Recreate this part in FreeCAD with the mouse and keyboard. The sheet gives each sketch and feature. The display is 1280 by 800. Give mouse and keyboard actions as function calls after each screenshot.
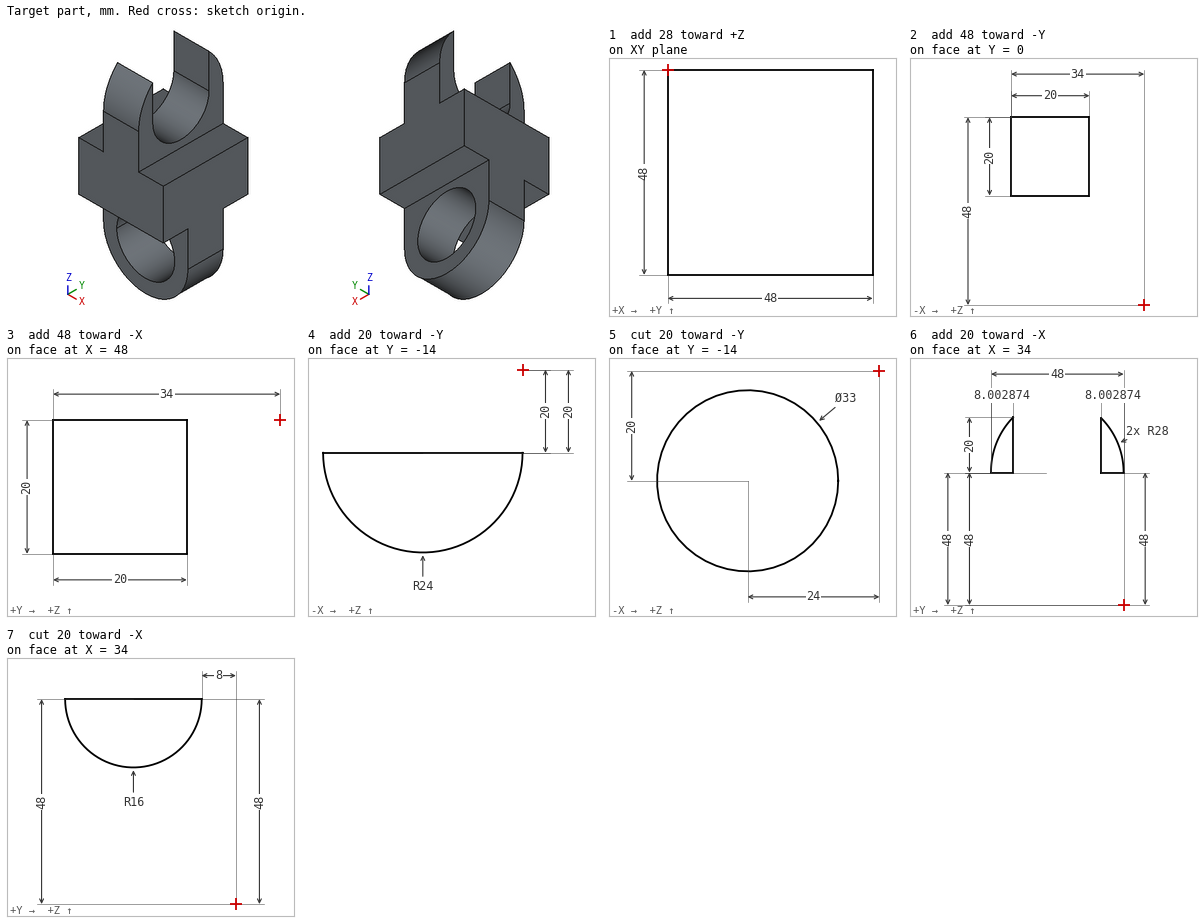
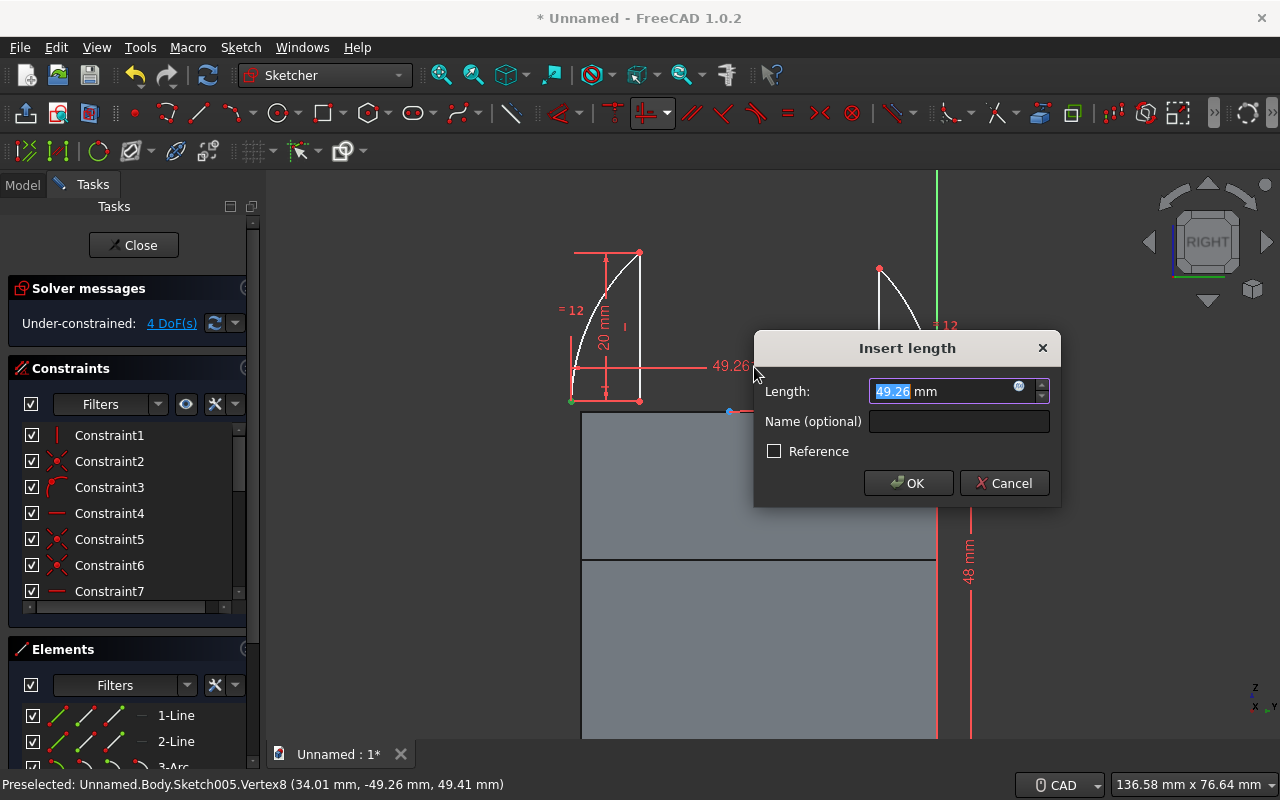
text(48)
key(Return)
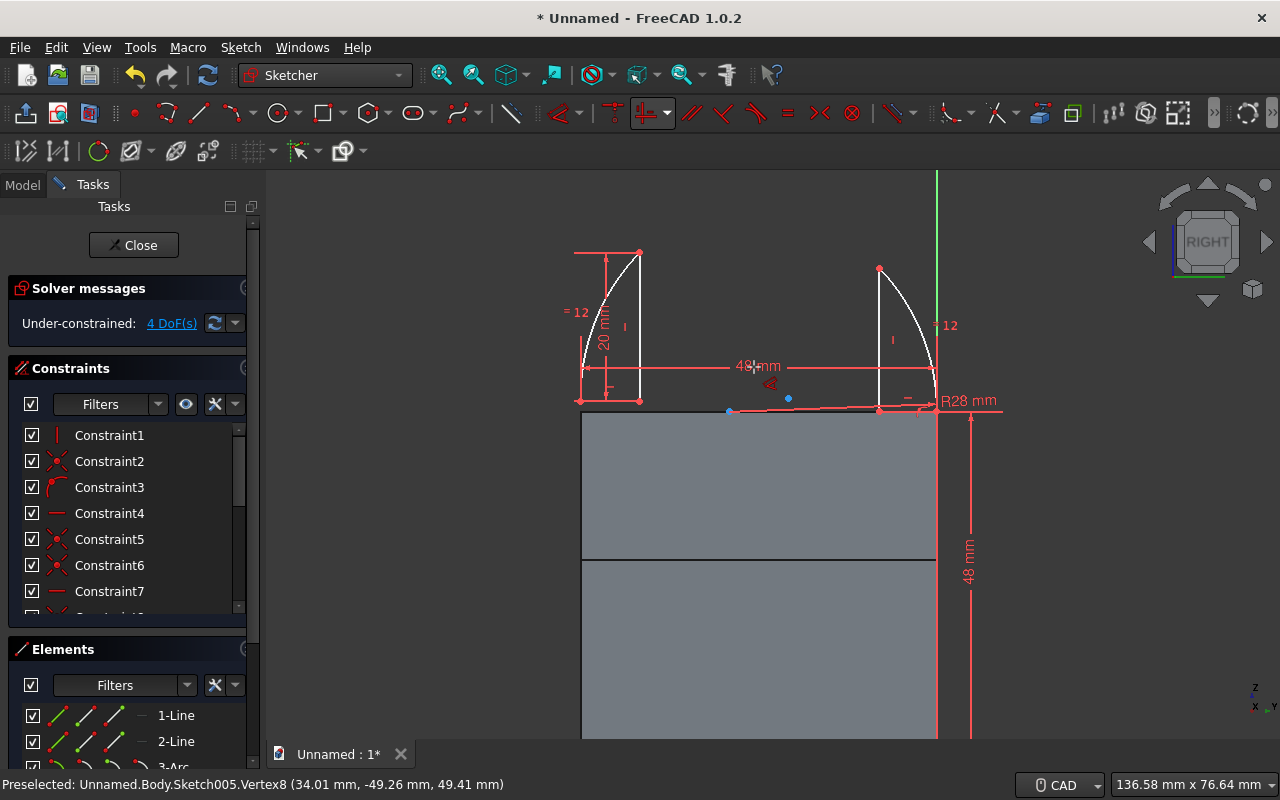
click(581, 401)
click(971, 485)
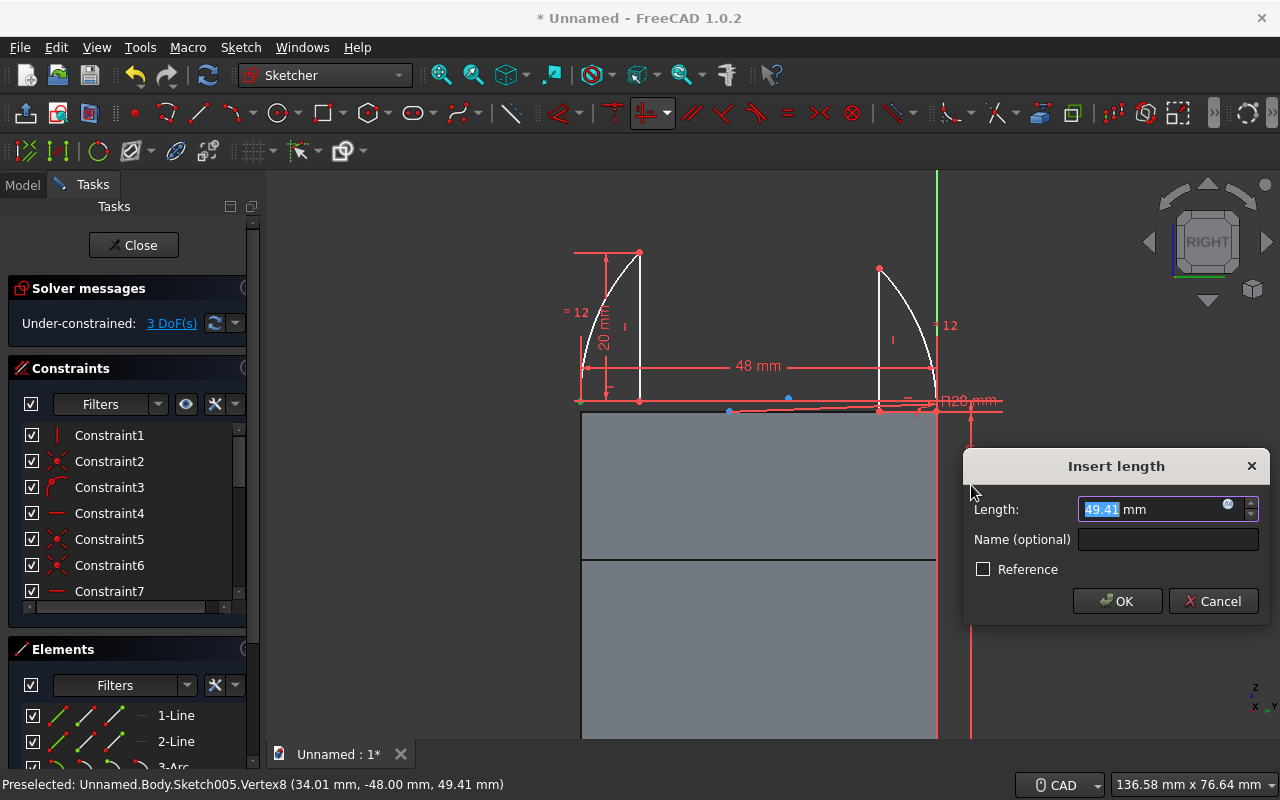
text(48)
key(Return)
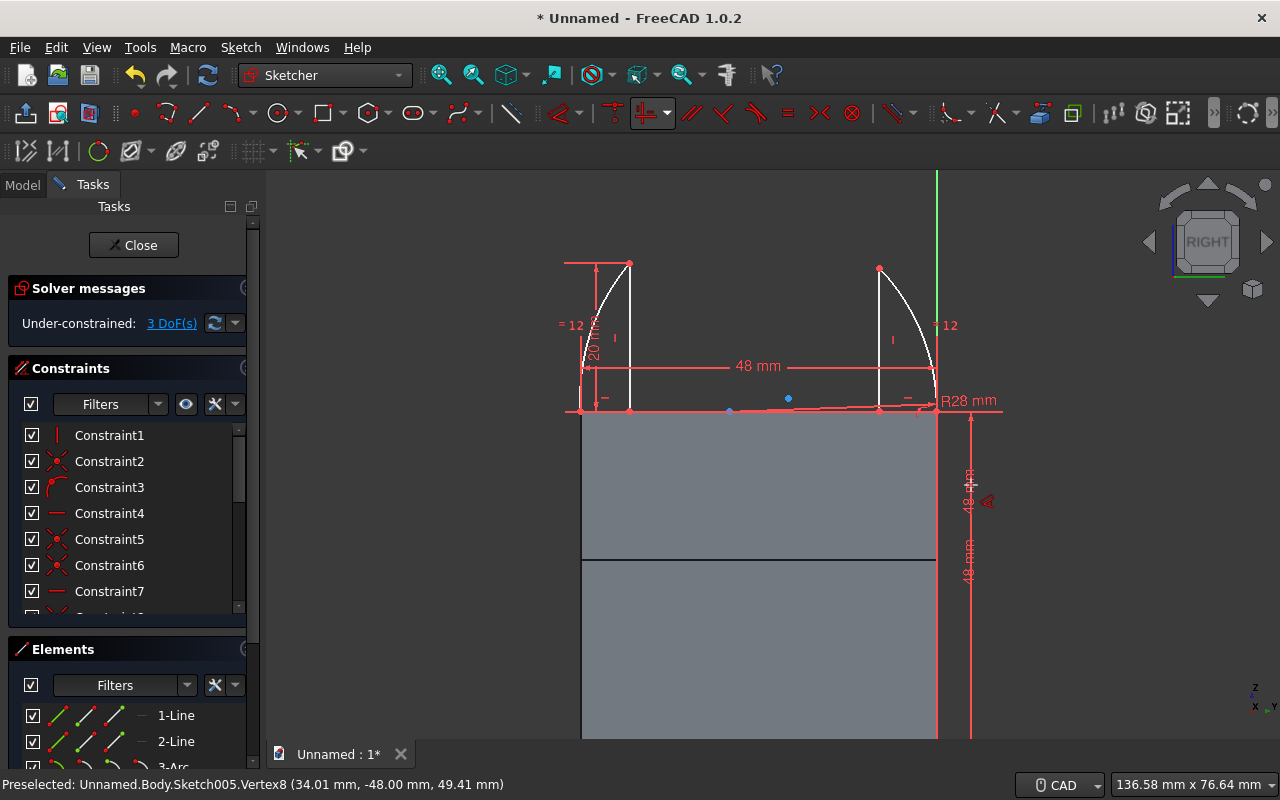
click(729, 412)
click(971, 630)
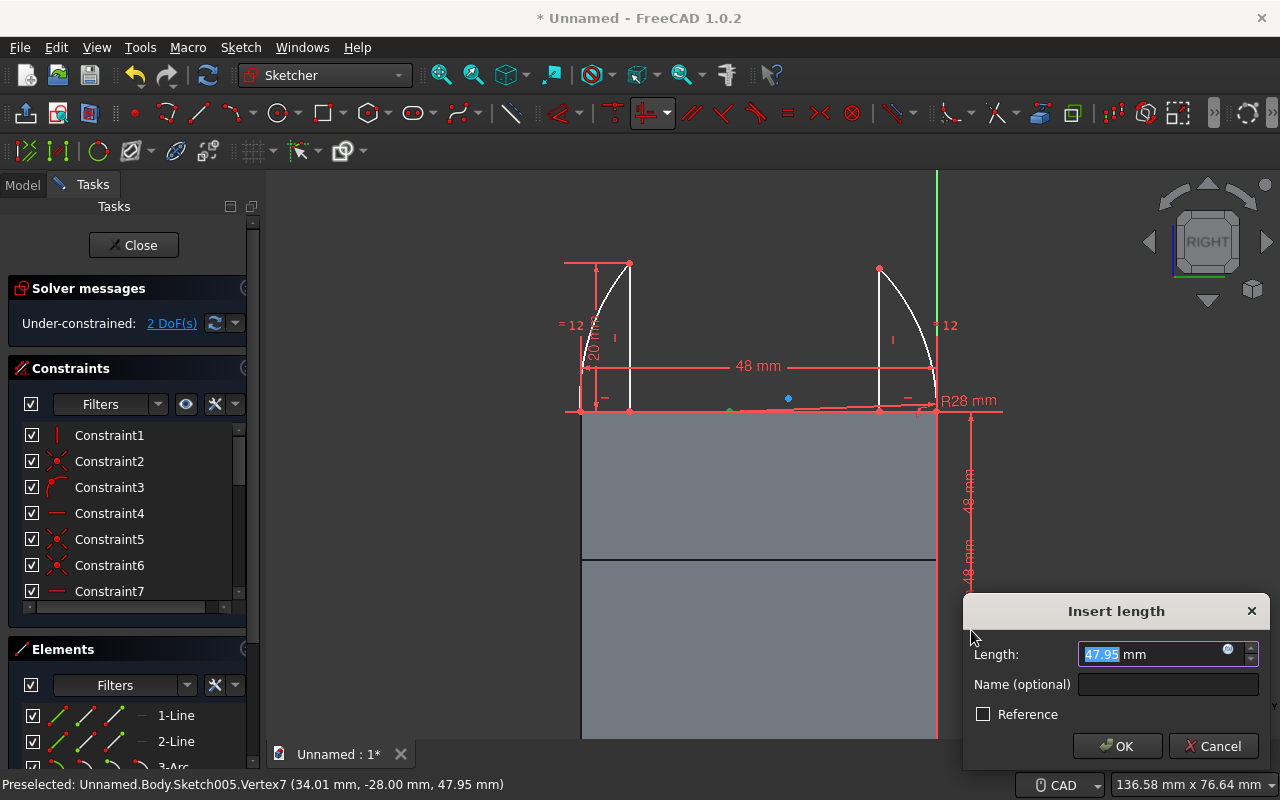
text(48)
key(Return)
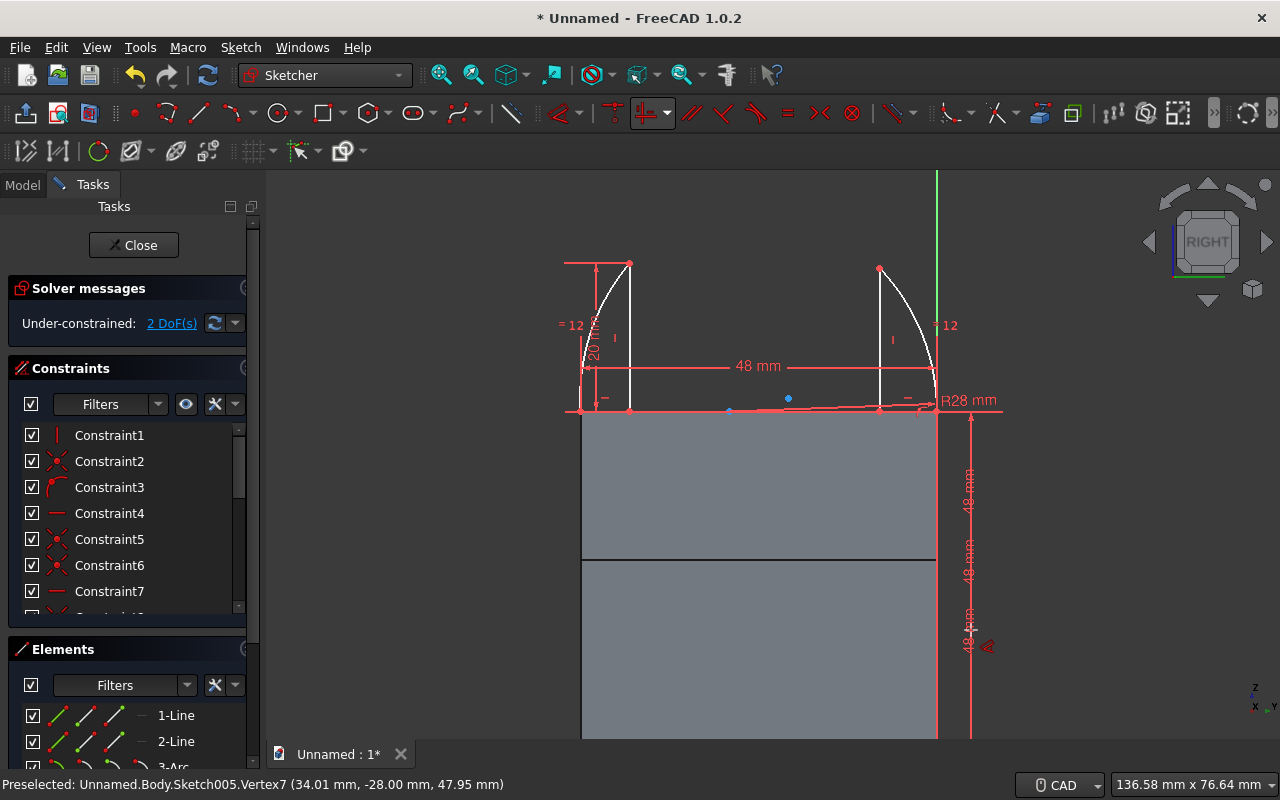
click(897, 412)
click(908, 378)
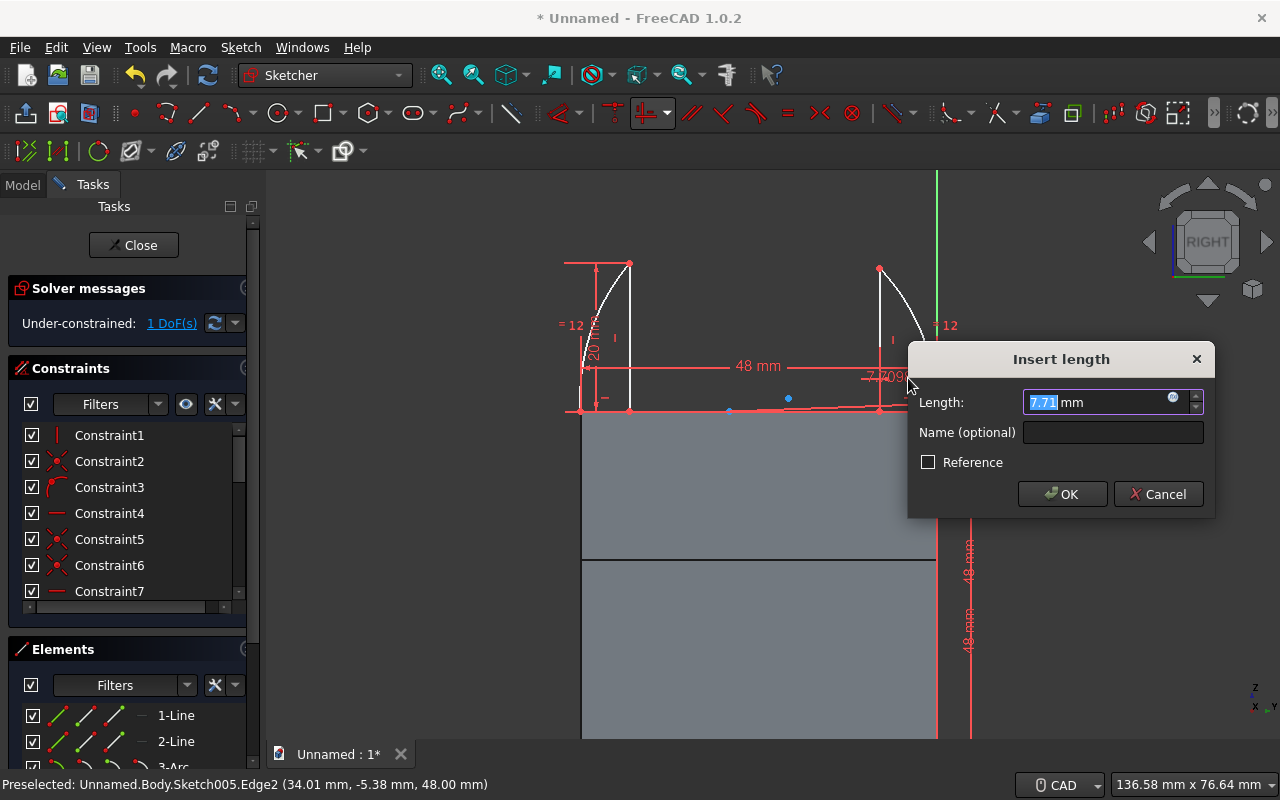
text(8.002874)
key(Return)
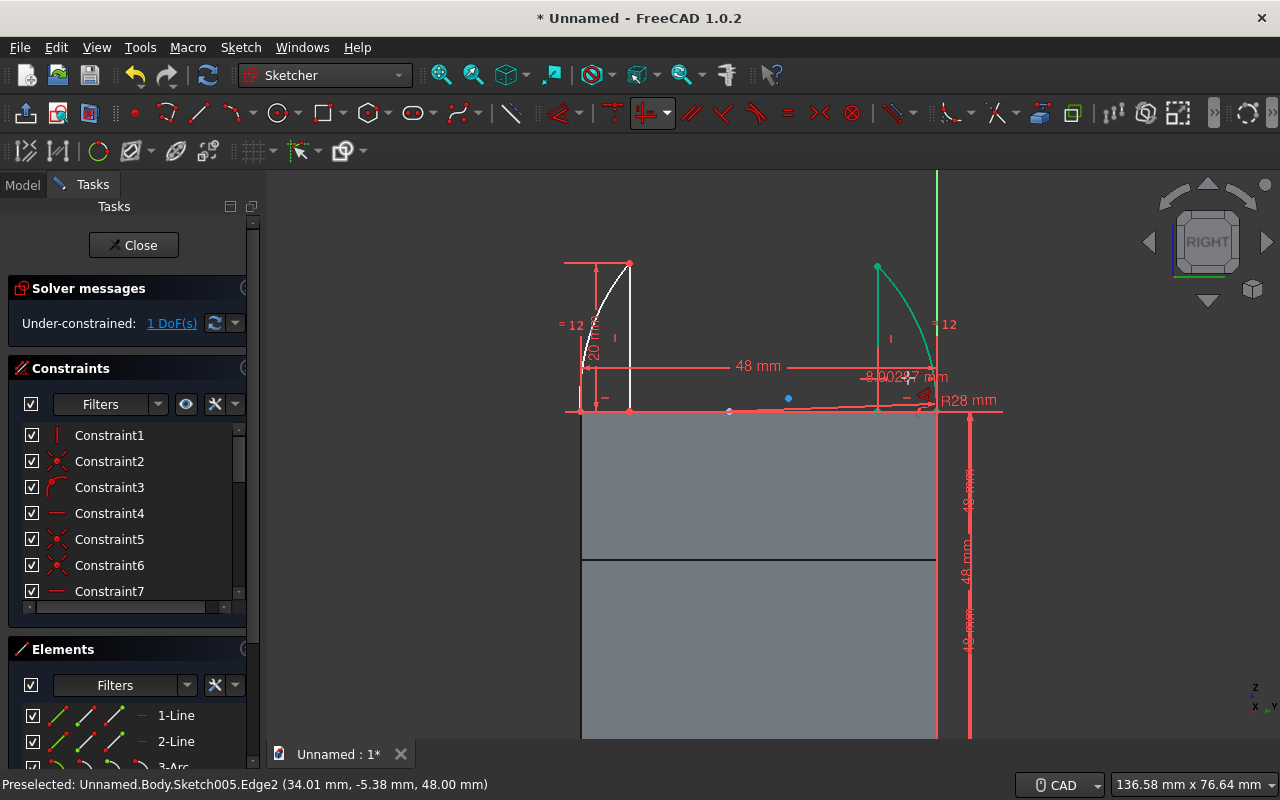
click(595, 412)
click(605, 378)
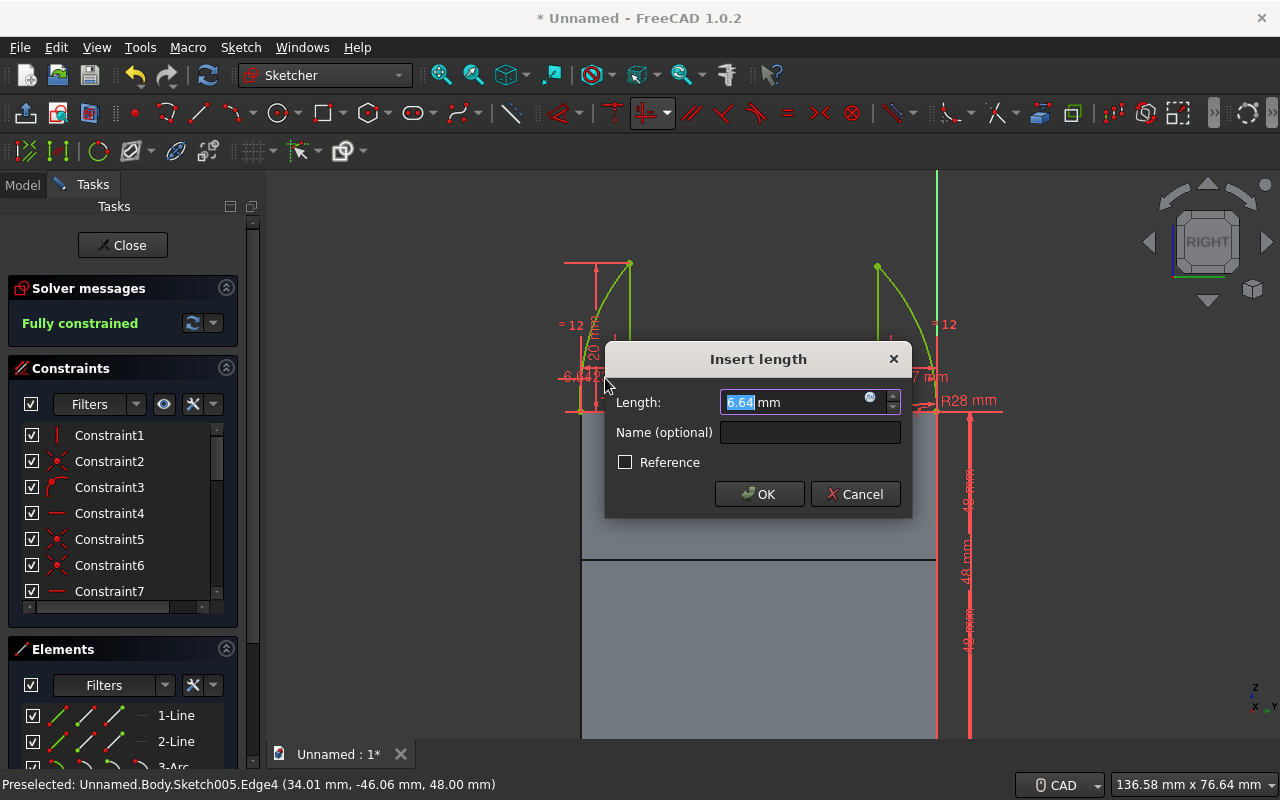
text(8.002874)
key(Return)
key(Escape)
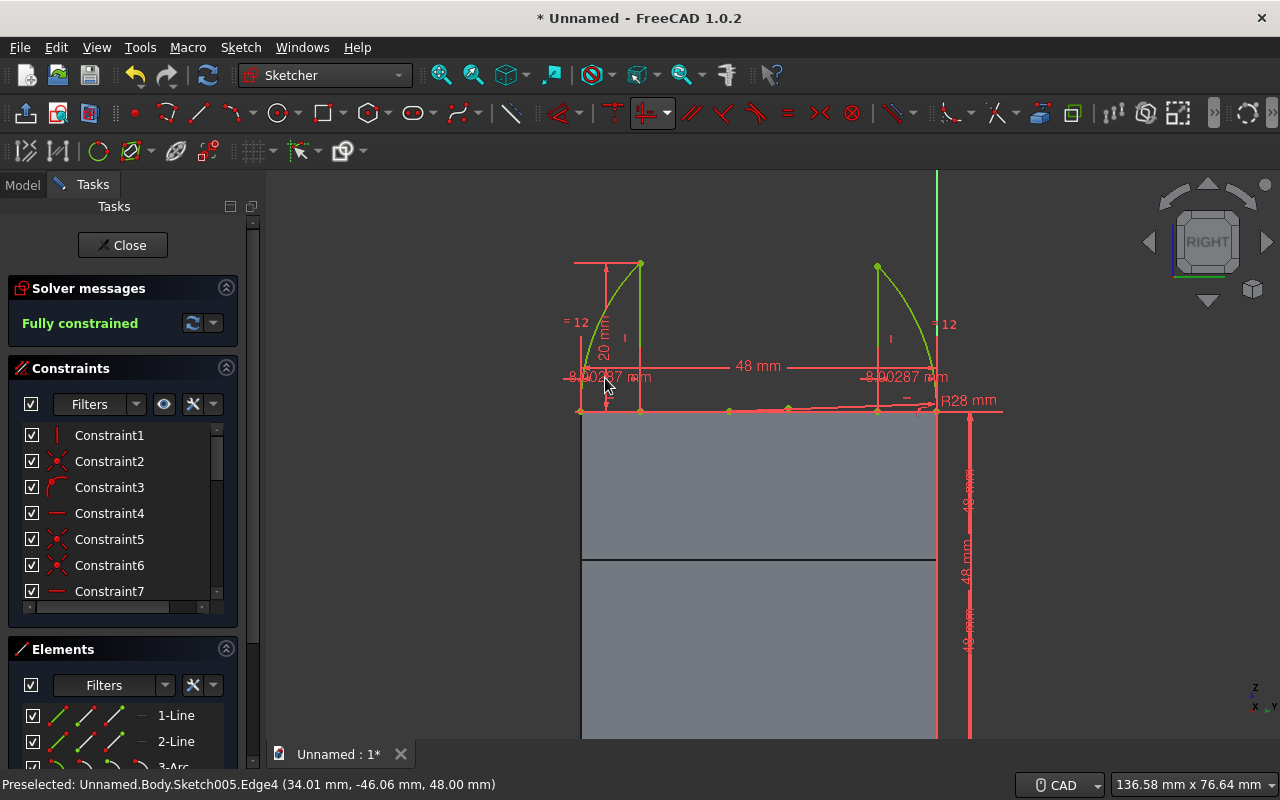
click(123, 245)